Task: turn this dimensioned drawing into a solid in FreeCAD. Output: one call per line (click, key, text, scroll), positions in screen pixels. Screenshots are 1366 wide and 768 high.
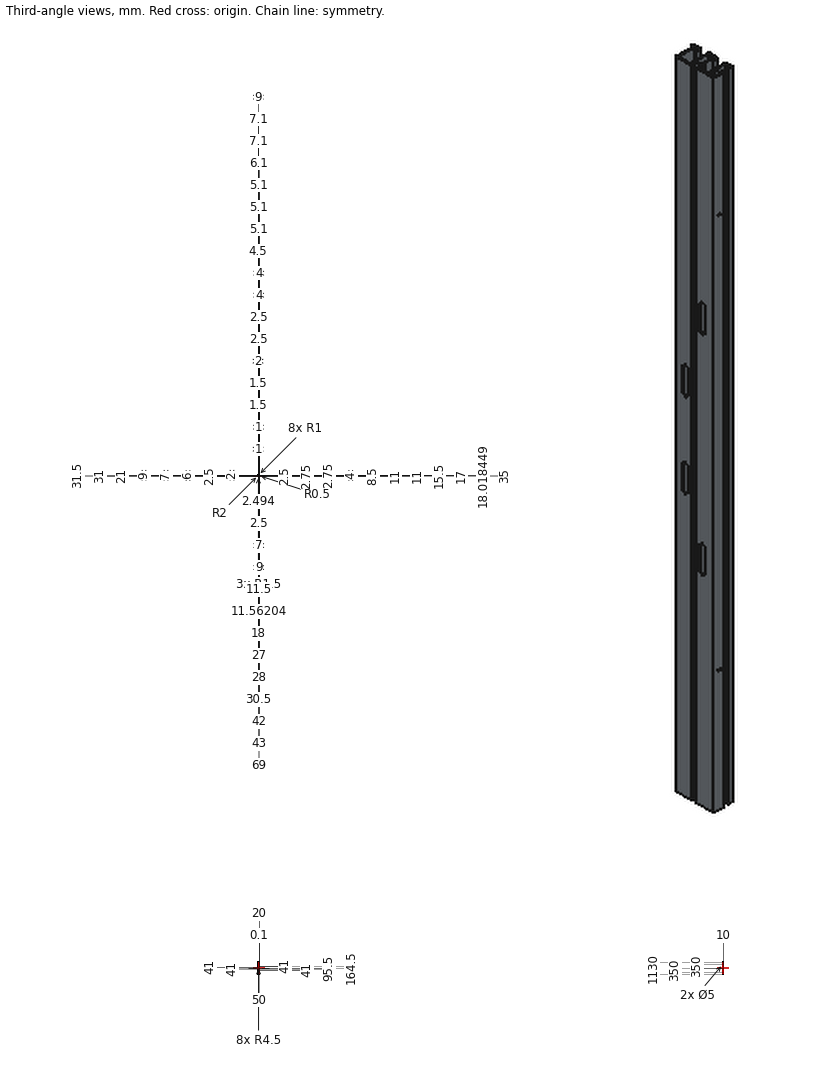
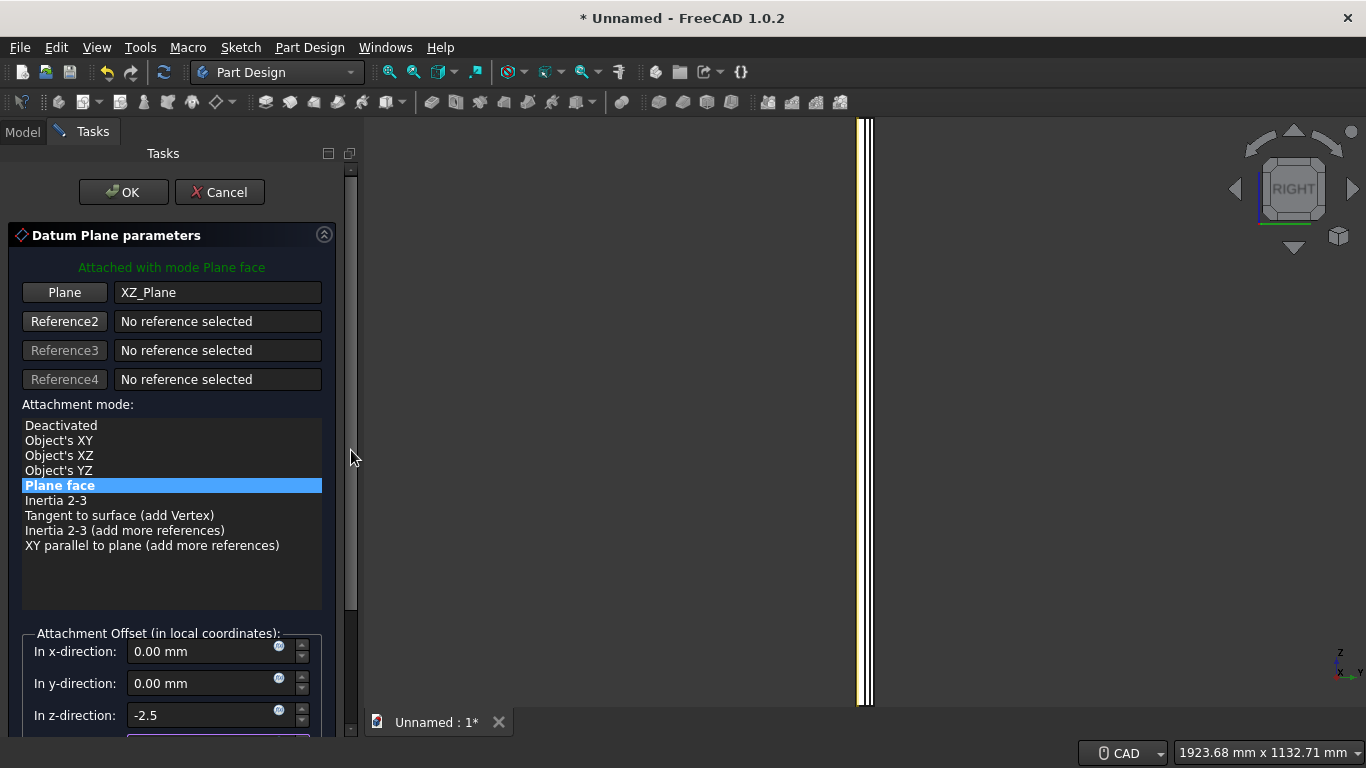
click(124, 192)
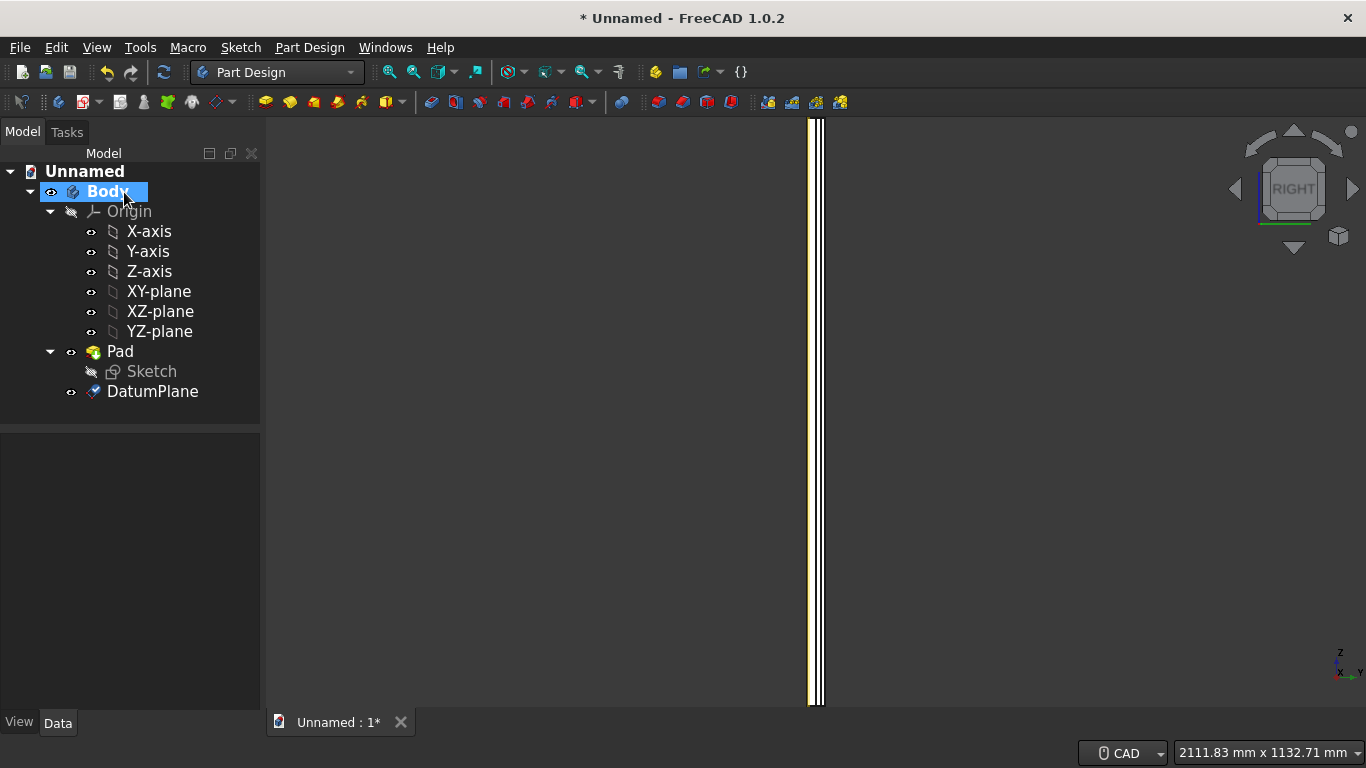
click(116, 392)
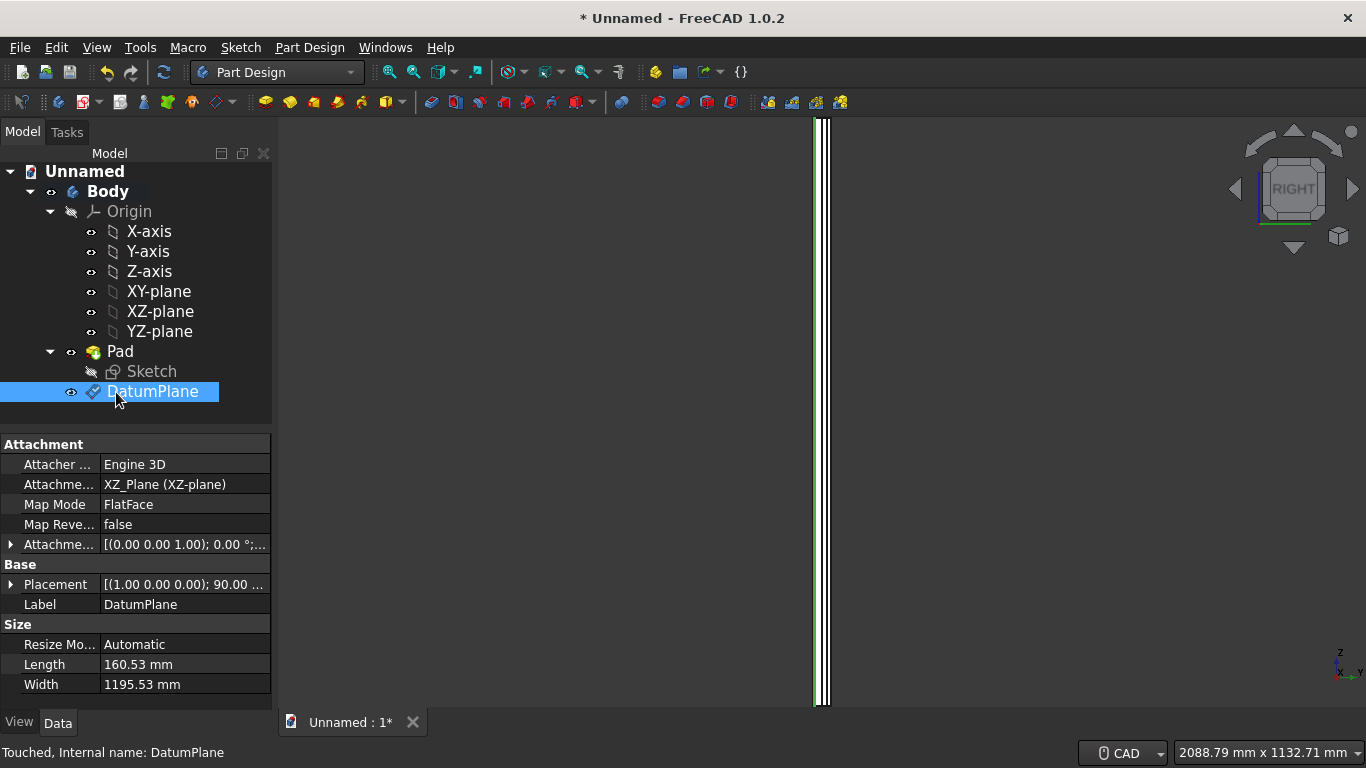
click(84, 102)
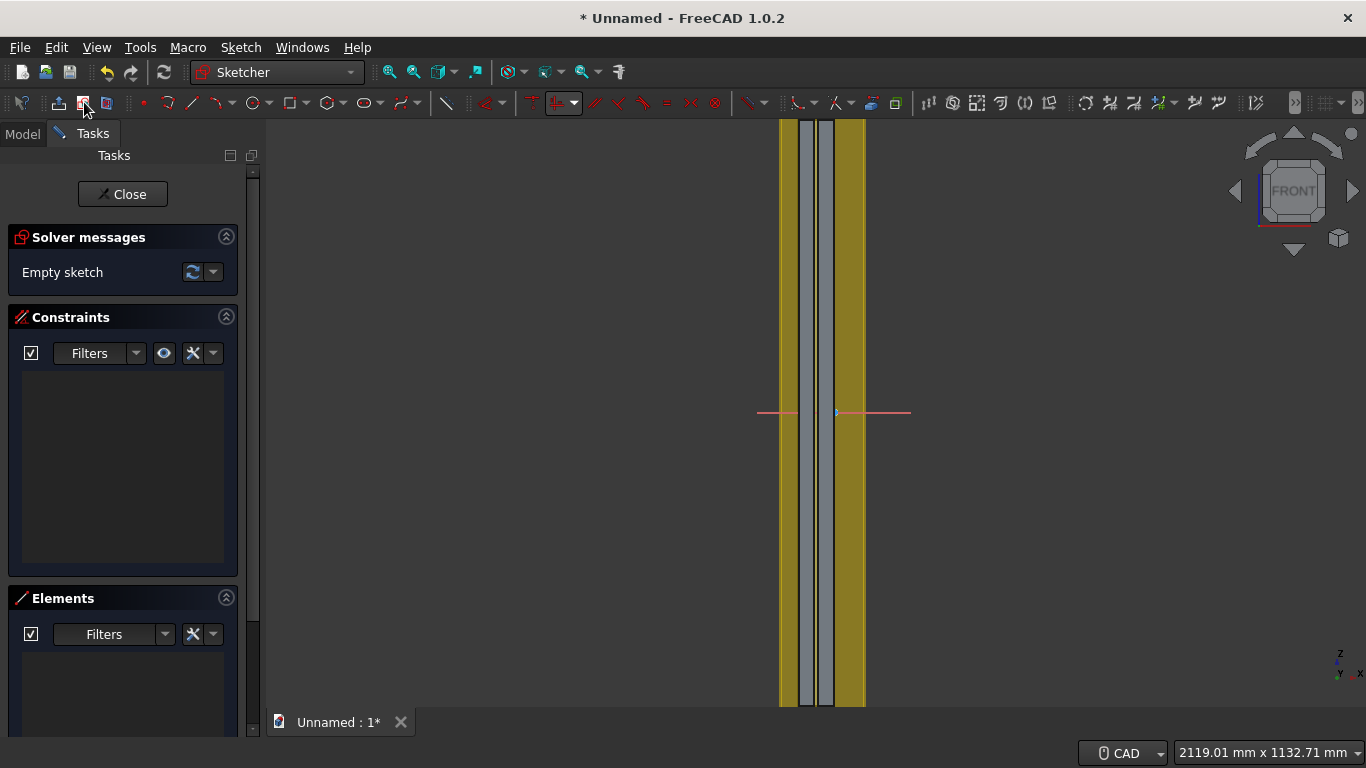
click(108, 104)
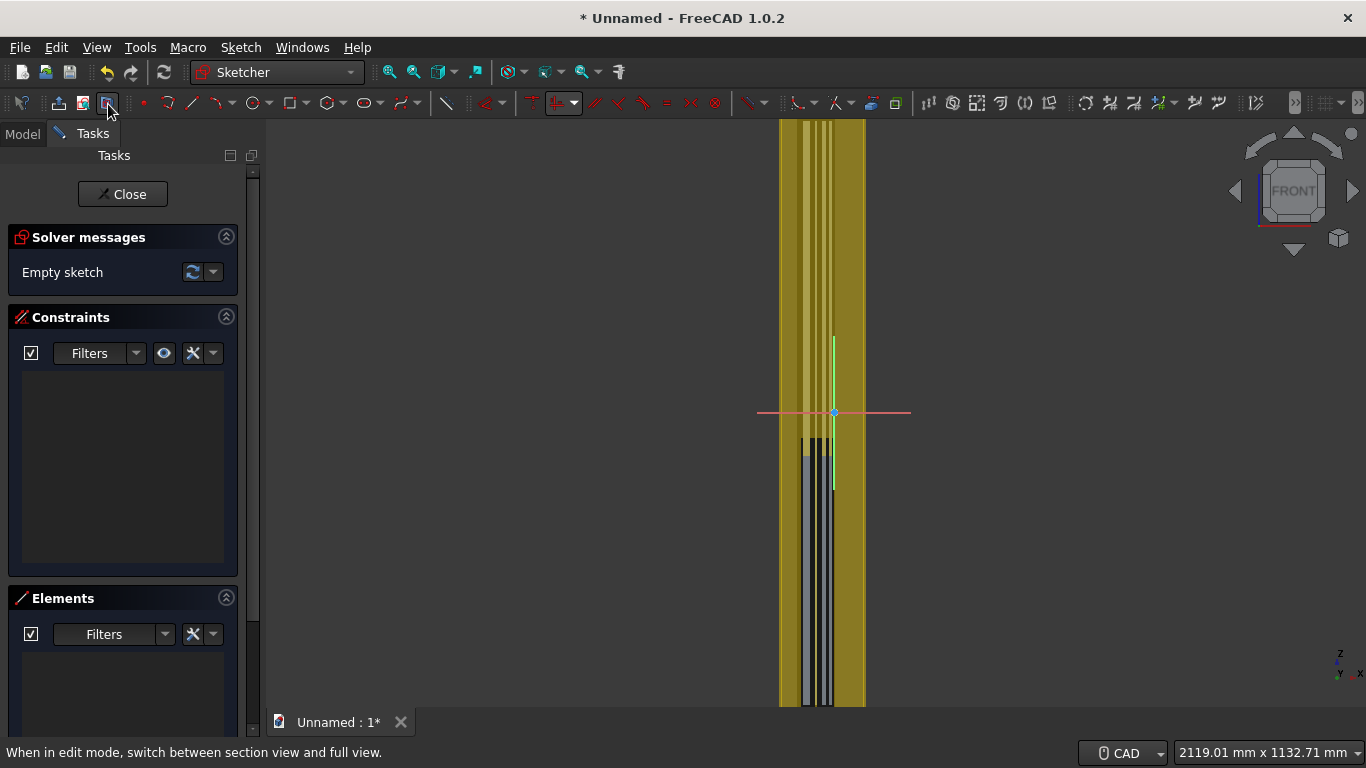
scroll(908, 413, up, 3)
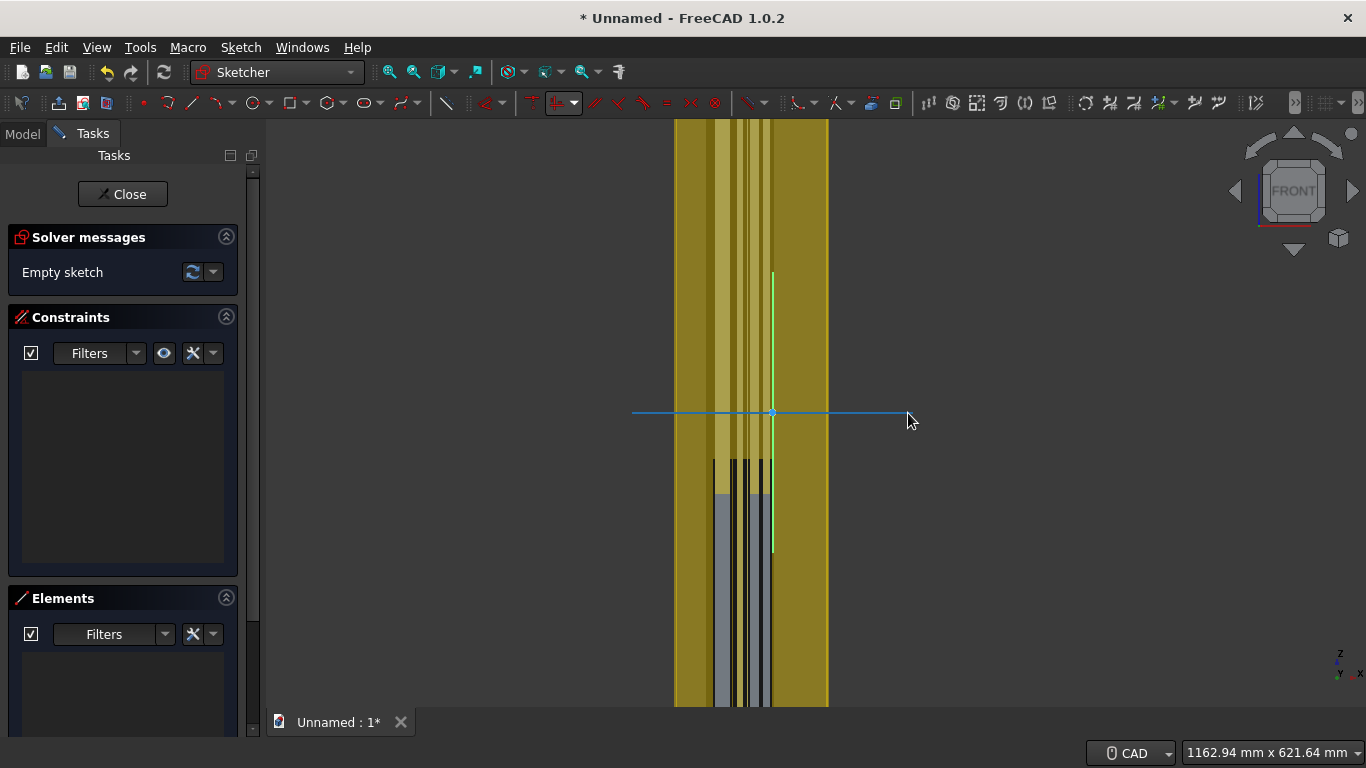
click(364, 104)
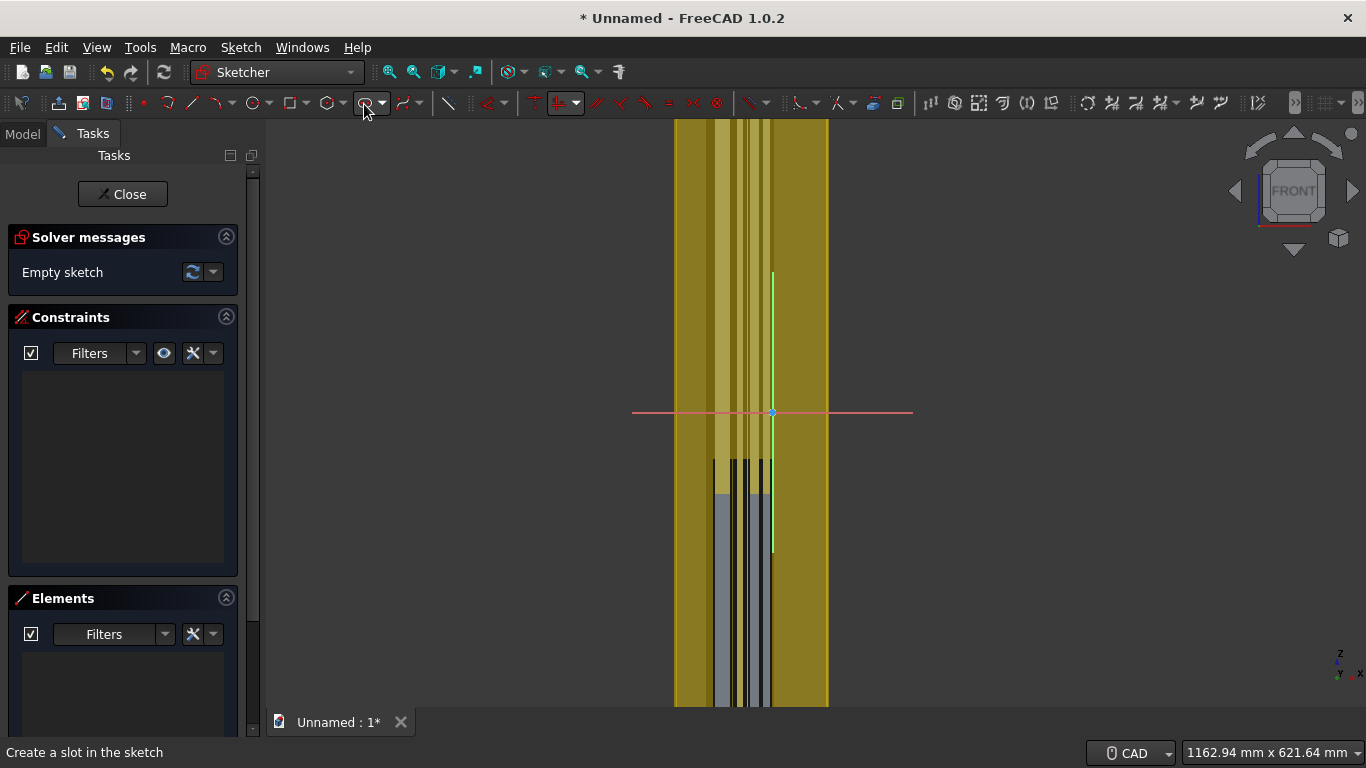
scroll(754, 257, up, 9)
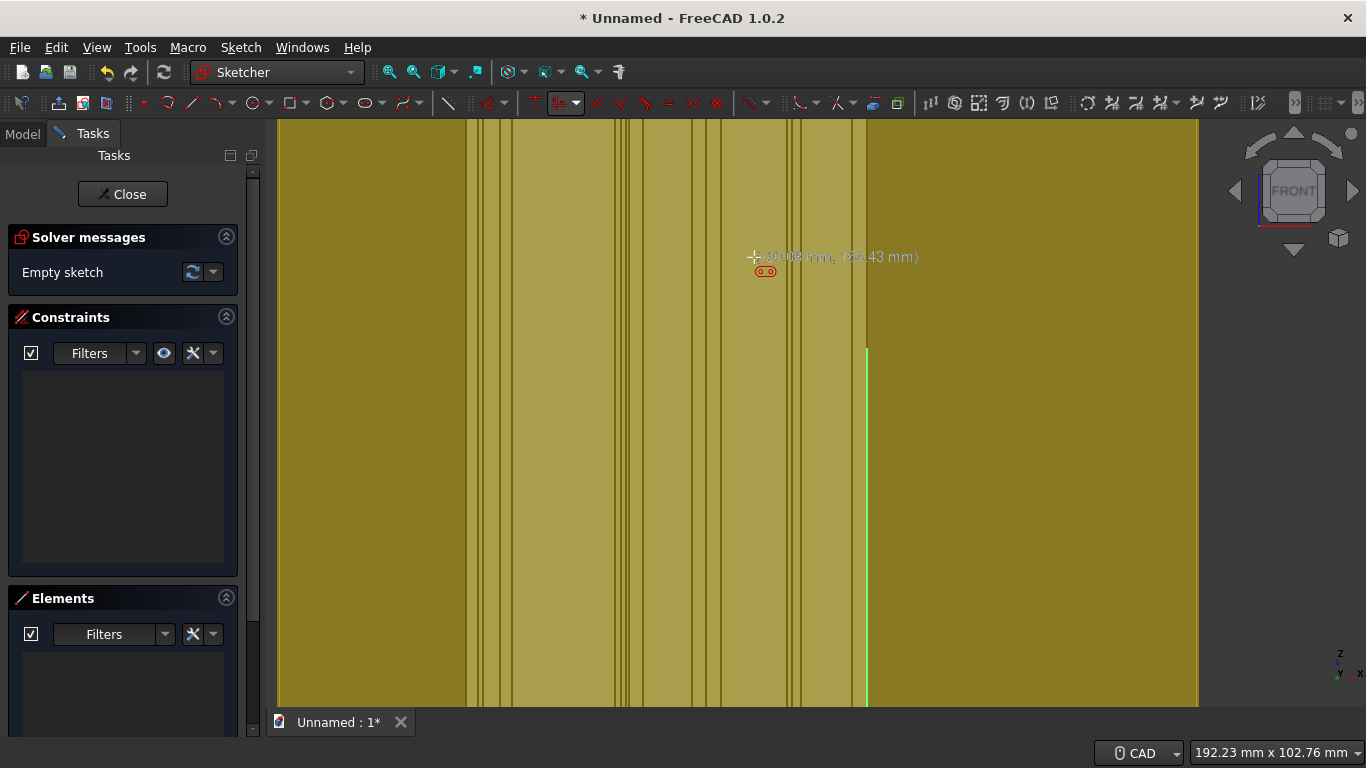
scroll(755, 258, down, 9)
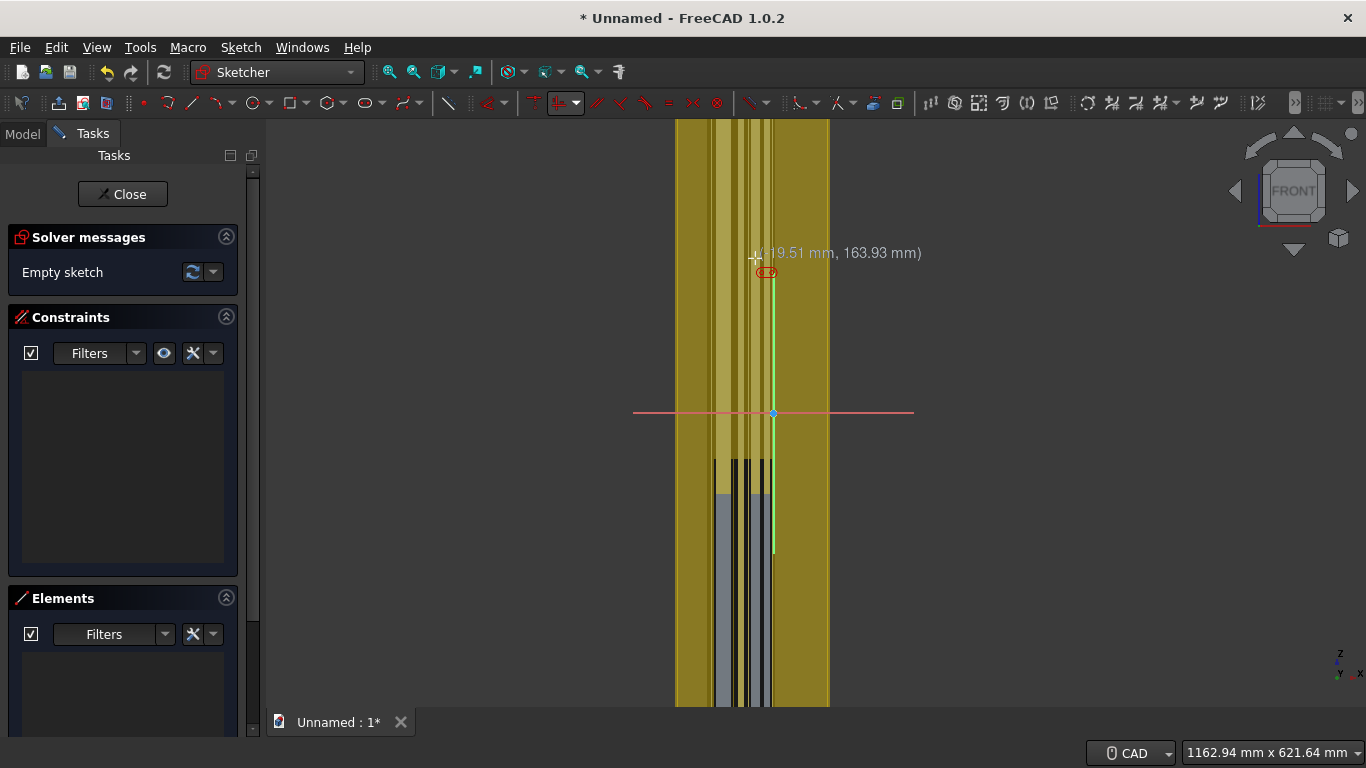
click(755, 258)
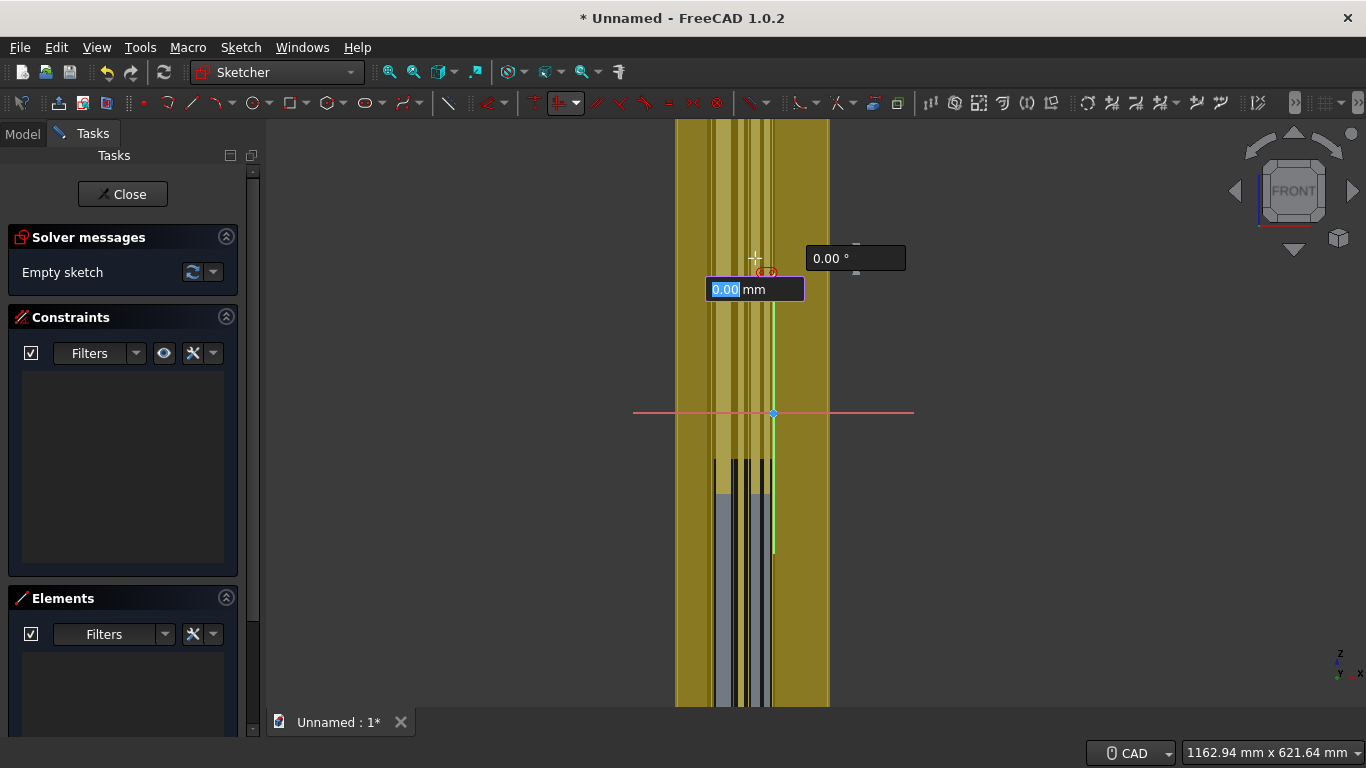
click(755, 219)